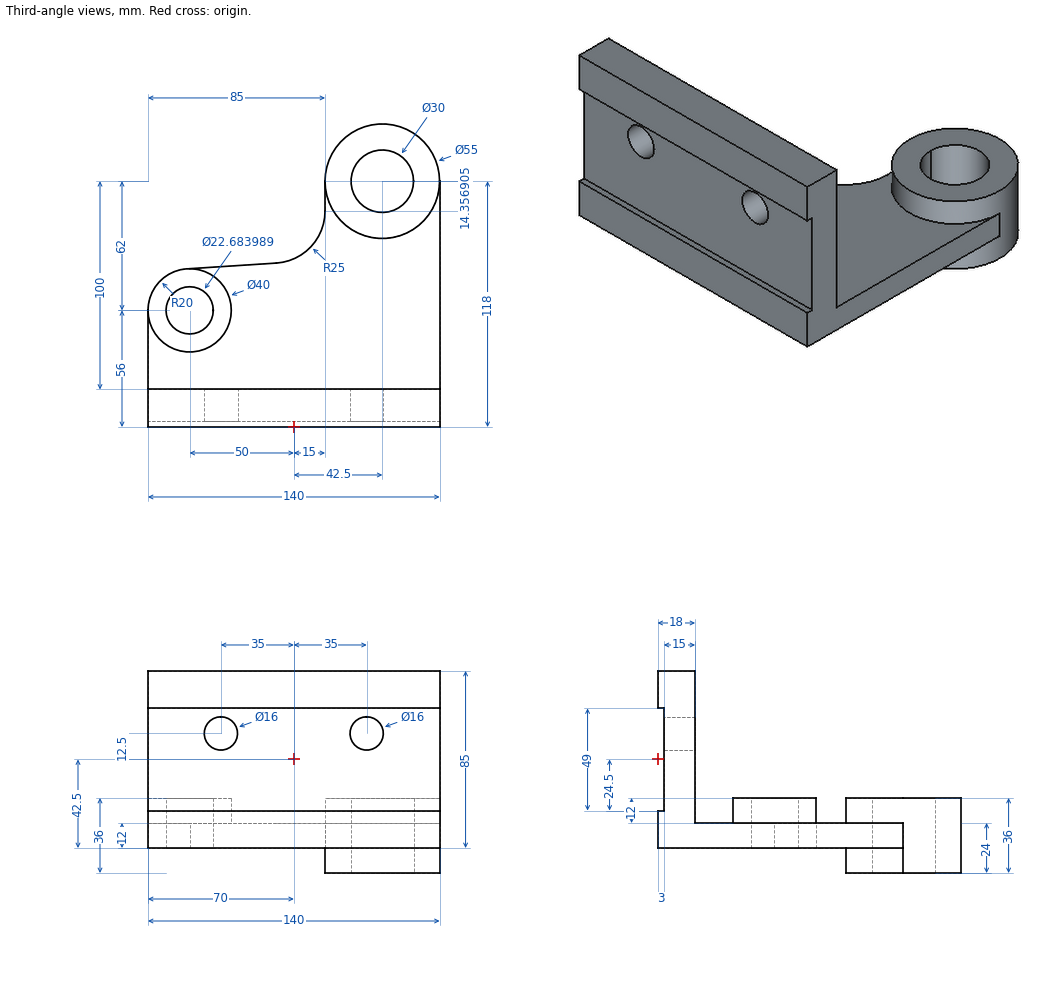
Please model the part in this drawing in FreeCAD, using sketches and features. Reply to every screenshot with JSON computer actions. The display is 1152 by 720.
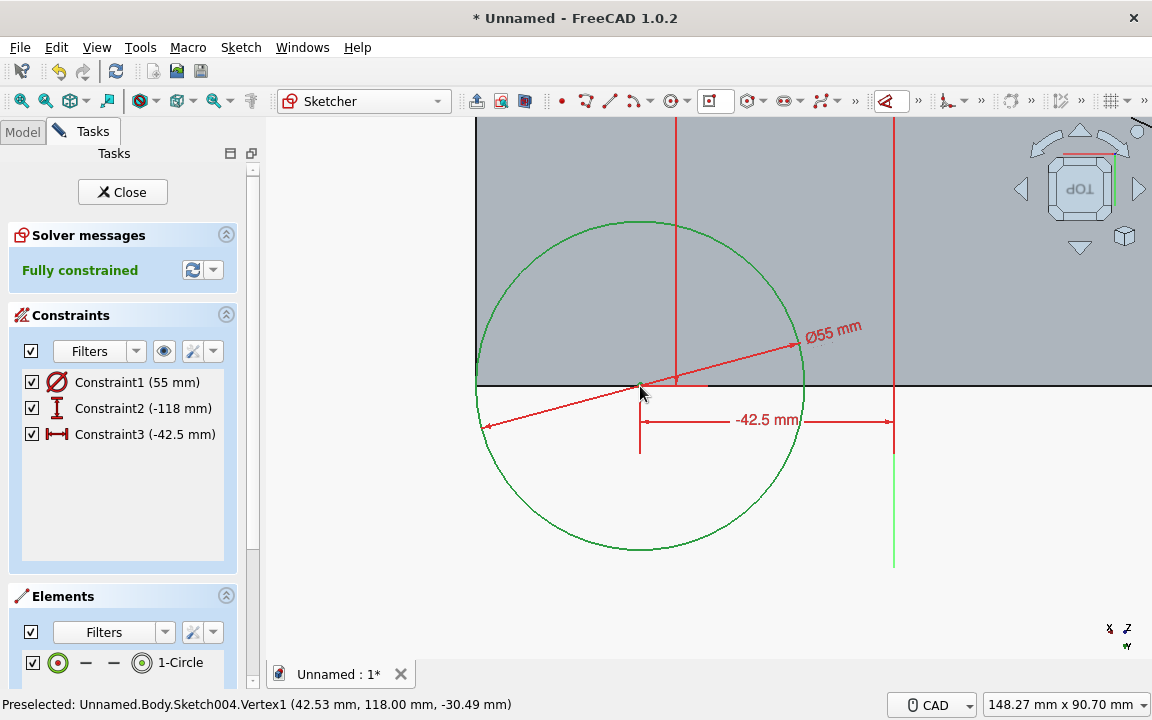
{"action": "left_click", "coordinate": [123, 192]}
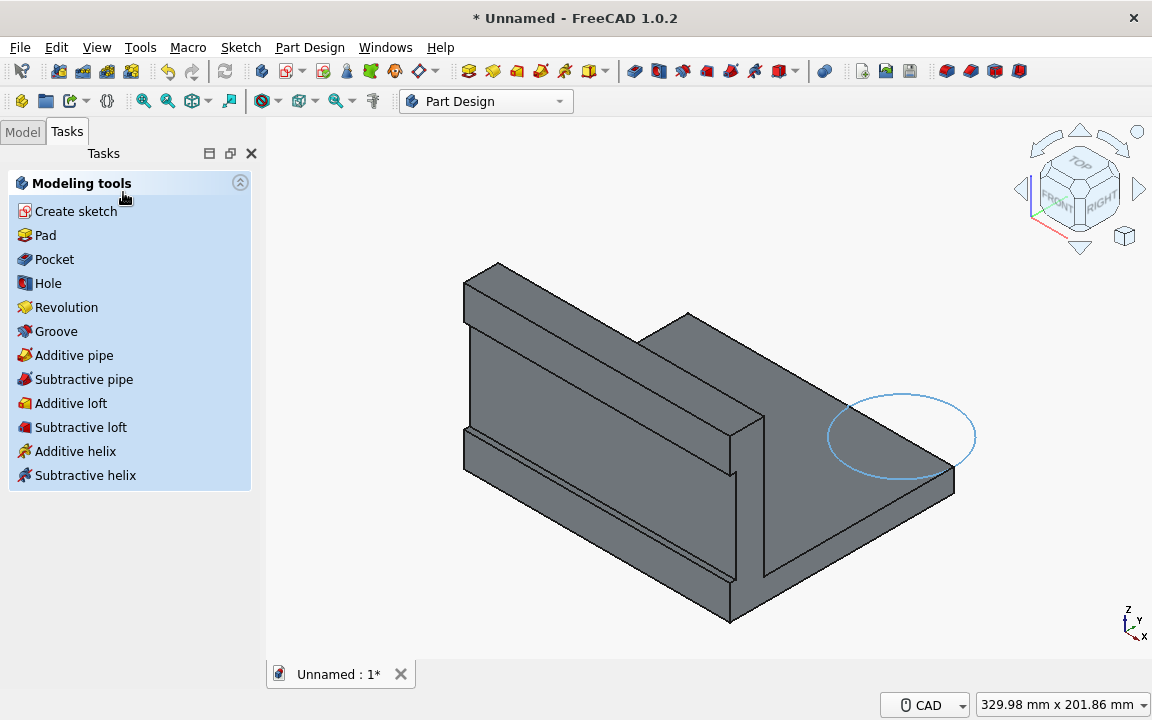
{"action": "left_click", "coordinate": [470, 72]}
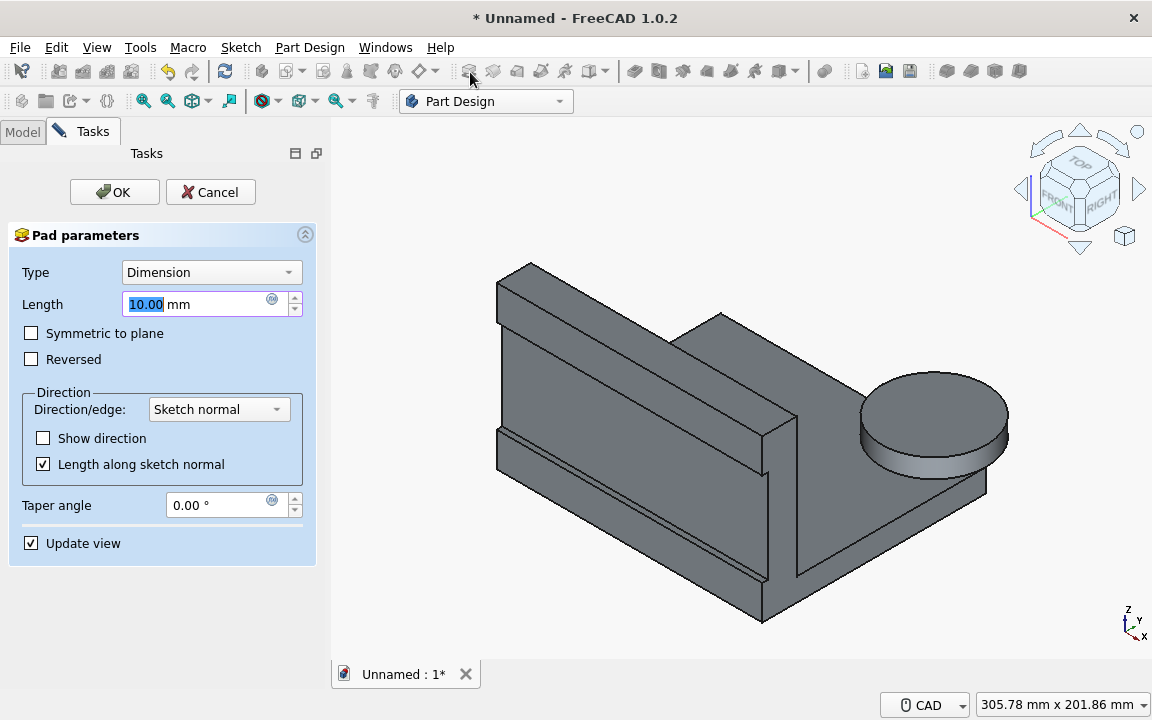
{"action": "type", "text": "24"}
{"action": "key", "text": "Tab"}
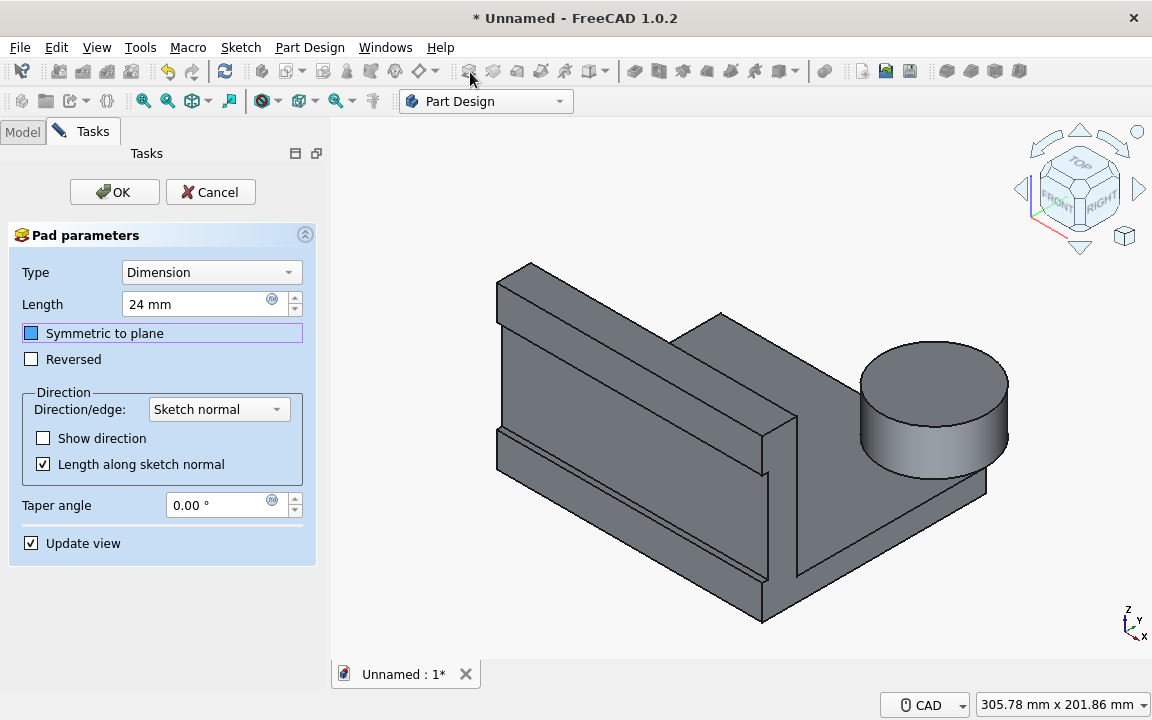
{"action": "left_click", "coordinate": [30, 359]}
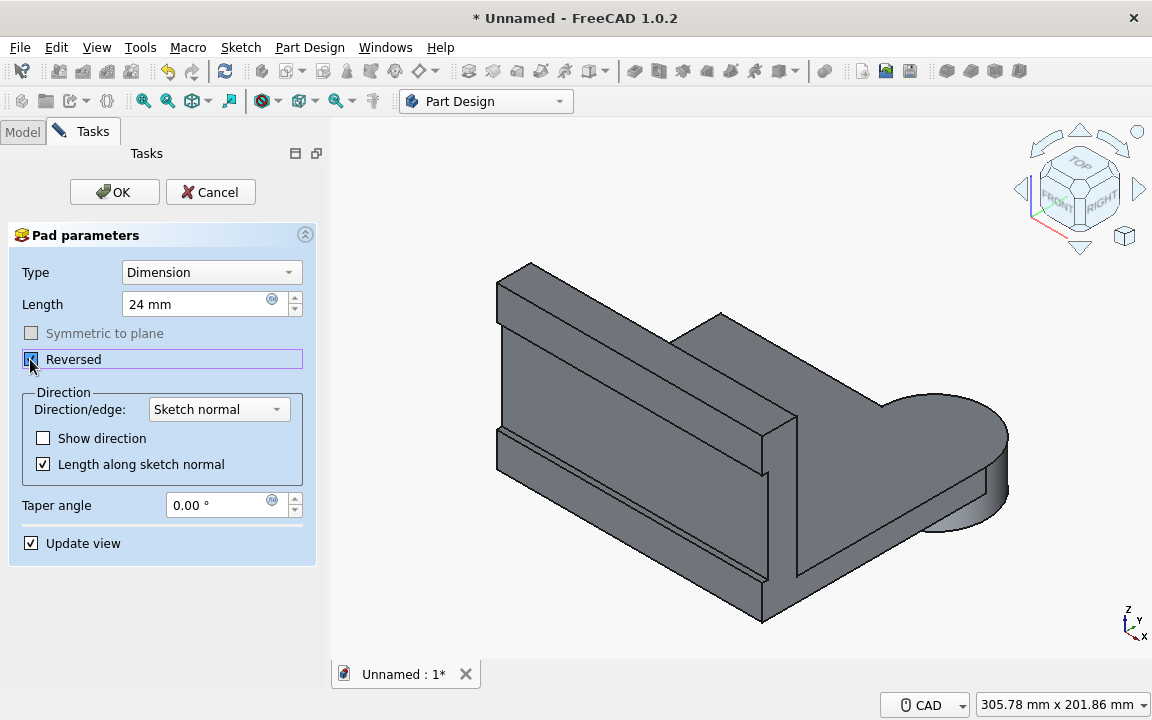
{"action": "left_click", "coordinate": [115, 192]}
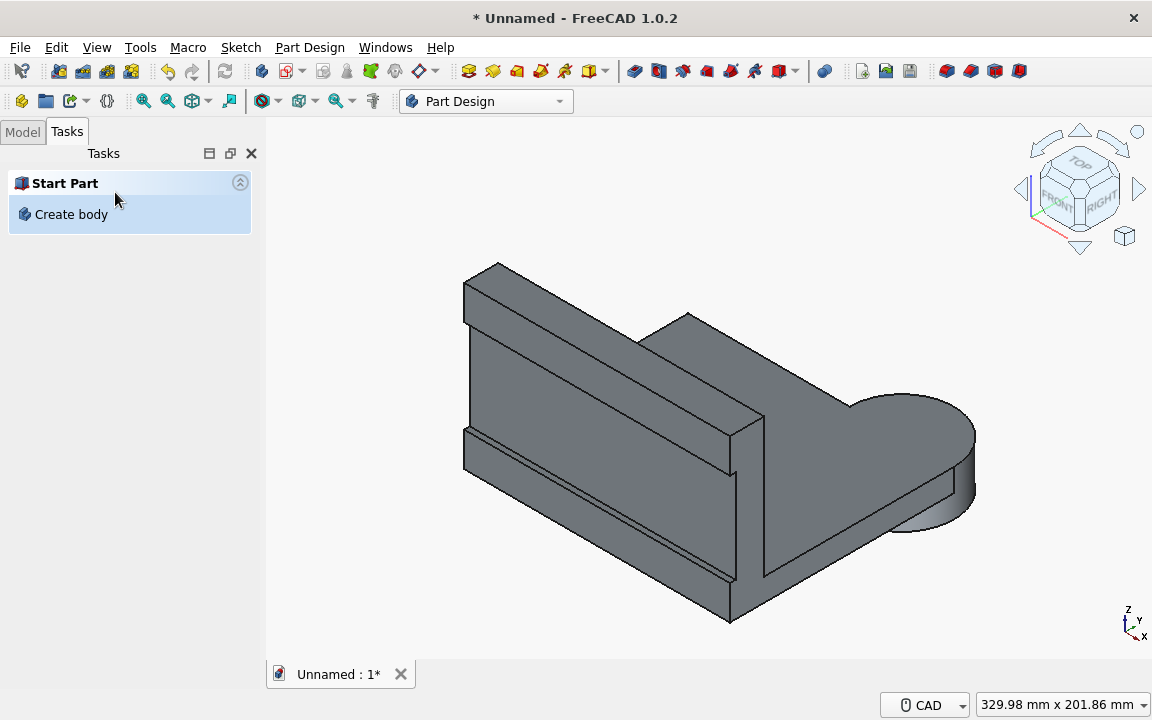
{"action": "key", "text": "2"}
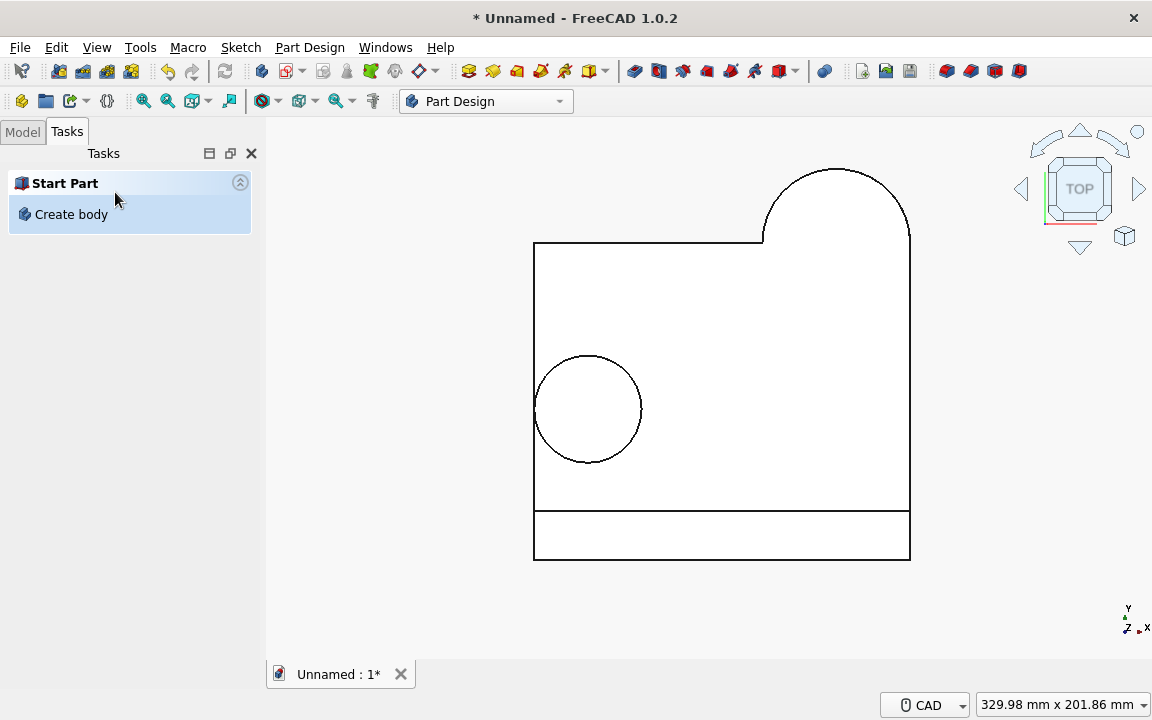
{"action": "left_click", "coordinate": [588, 408]}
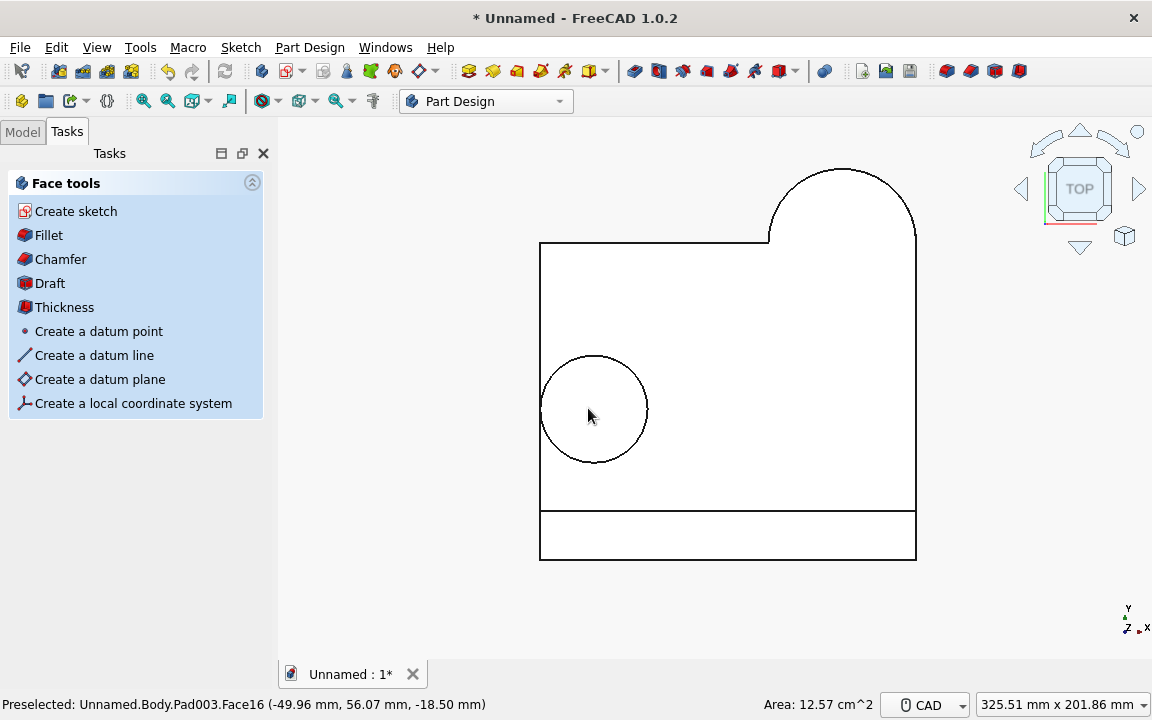
{"action": "left_click", "coordinate": [286, 72]}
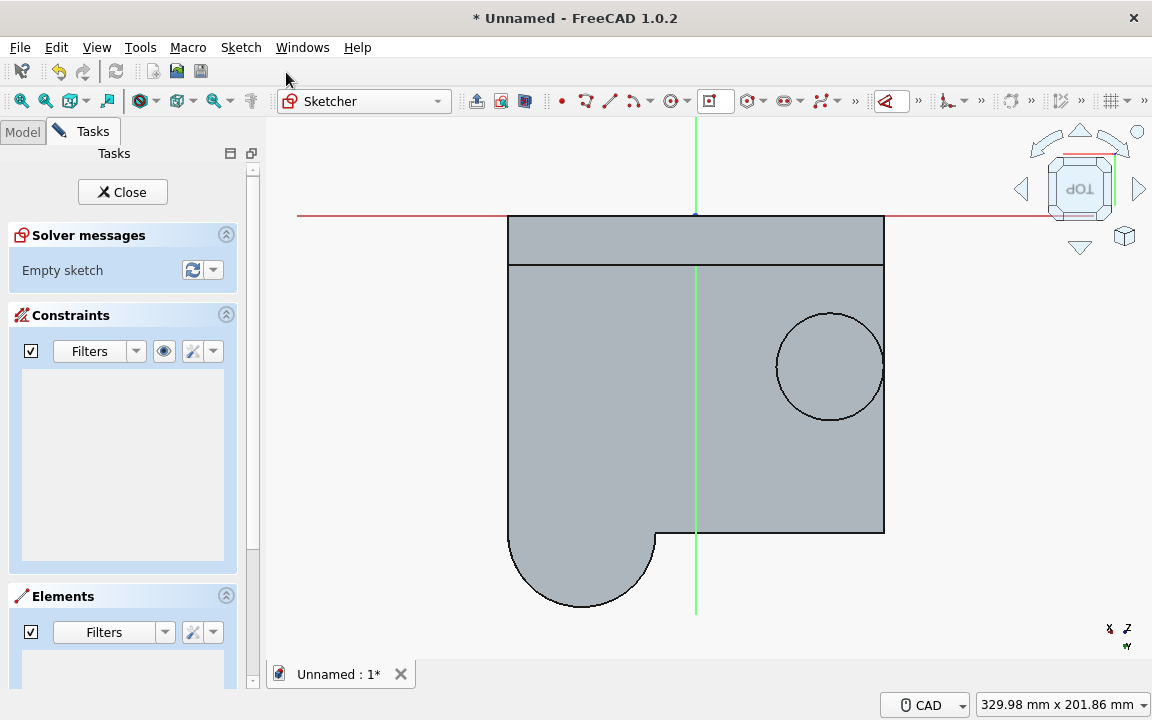
{"action": "scroll", "coordinate": [534, 631], "scroll_direction": "up", "scroll_amount": 4}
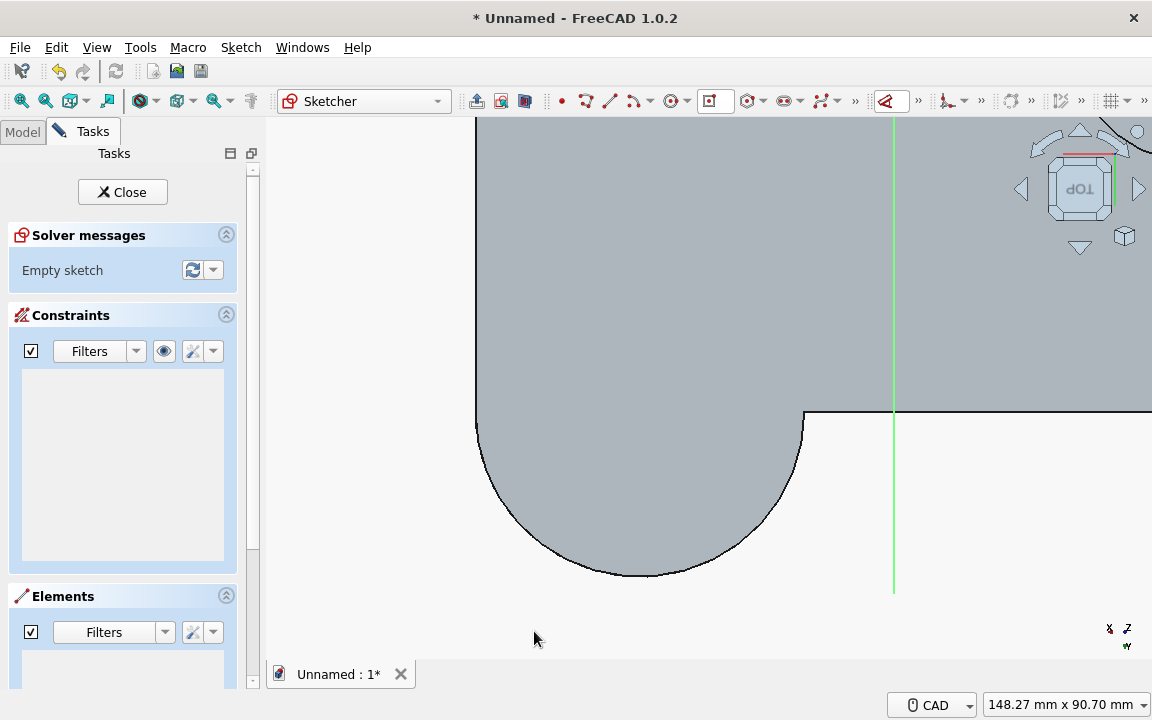
{"action": "left_click", "coordinate": [672, 102]}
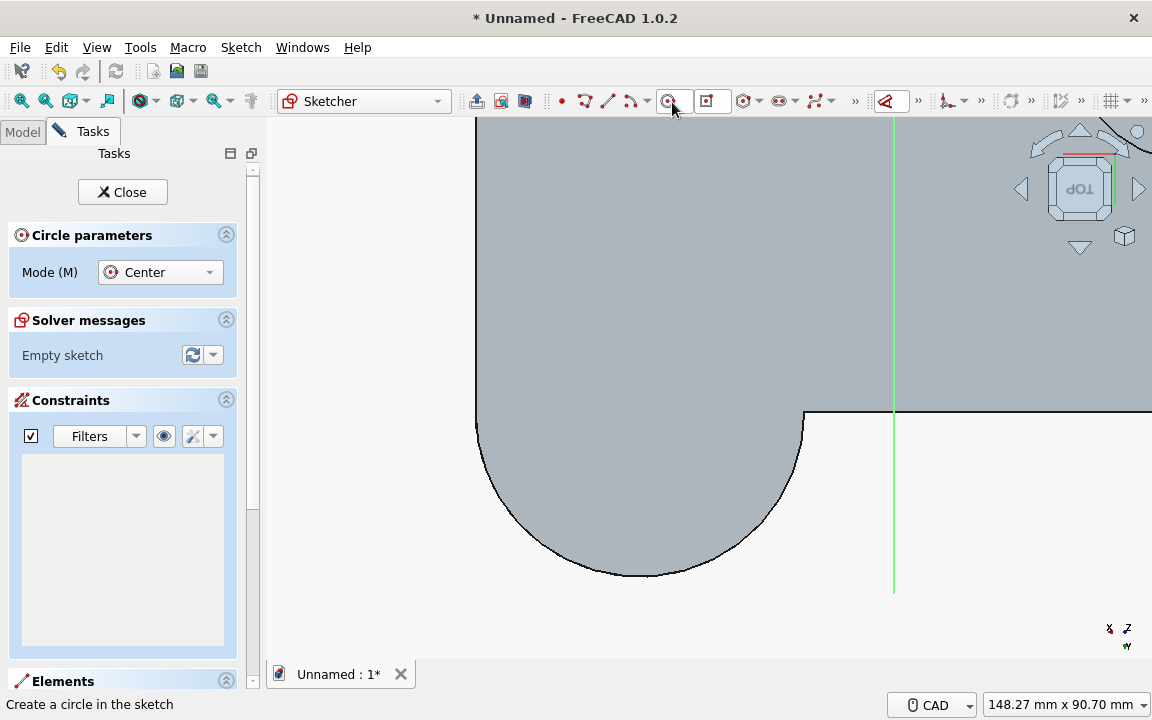
{"action": "left_click", "coordinate": [640, 412]}
{"action": "left_click", "coordinate": [756, 296]}
{"action": "key", "text": "Escape"}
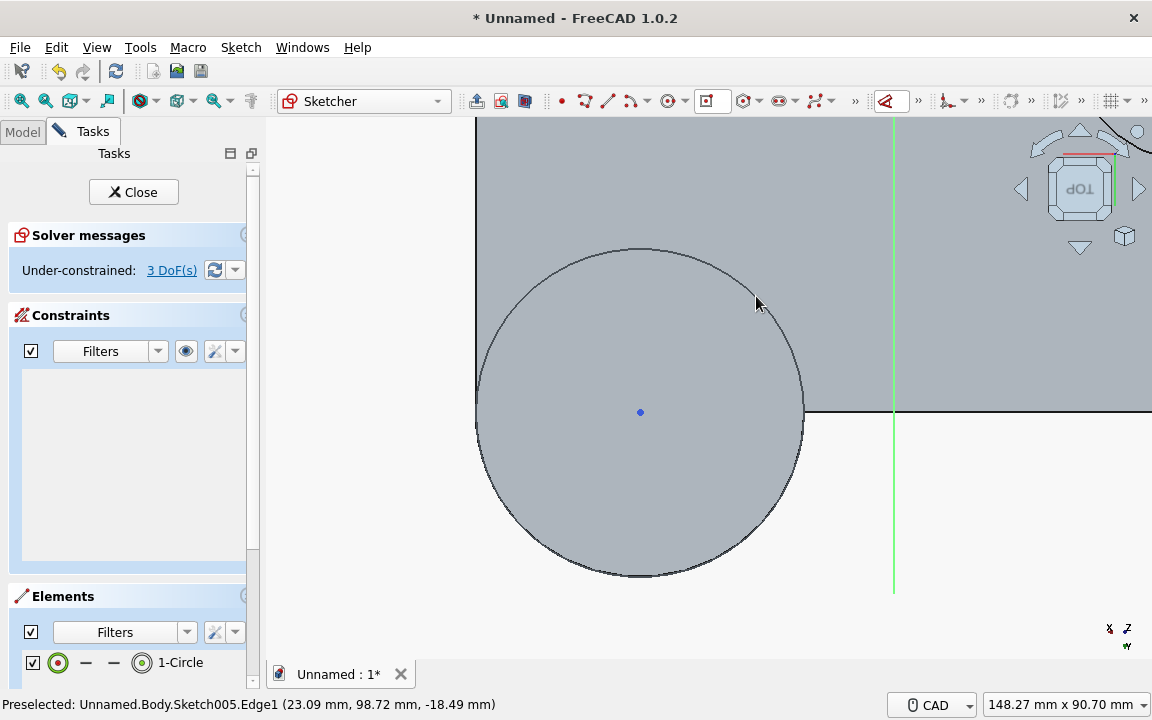
{"action": "left_click", "coordinate": [756, 297]}